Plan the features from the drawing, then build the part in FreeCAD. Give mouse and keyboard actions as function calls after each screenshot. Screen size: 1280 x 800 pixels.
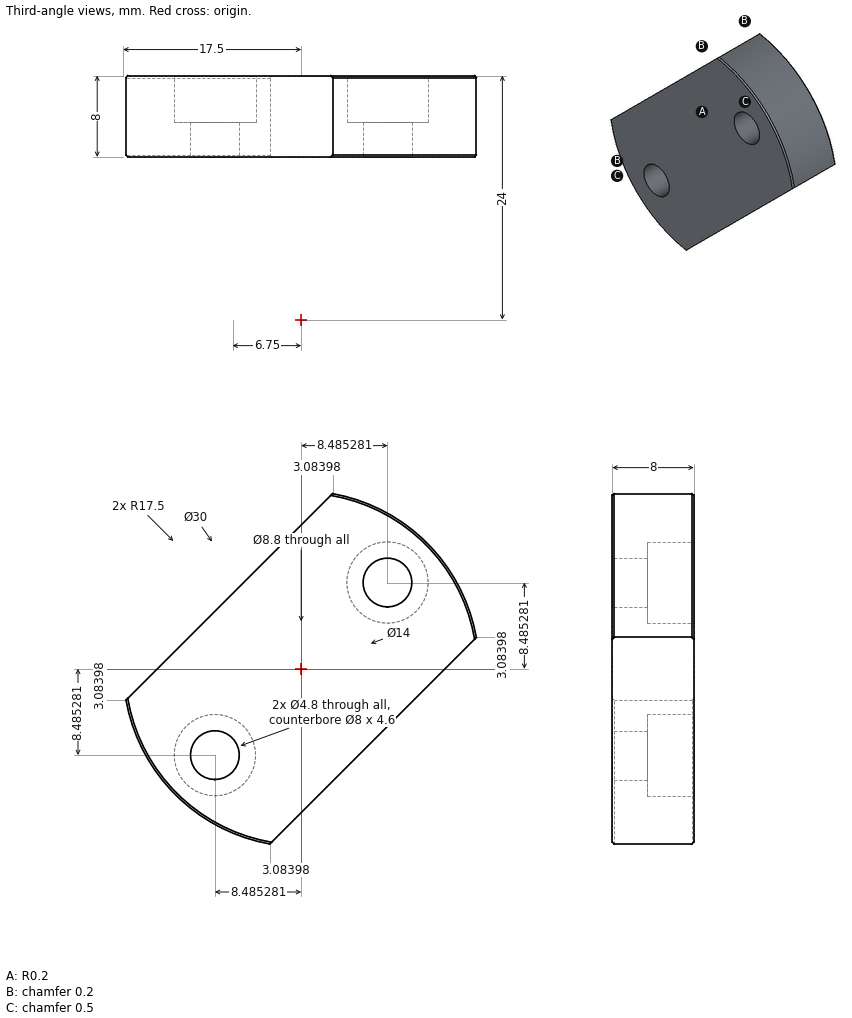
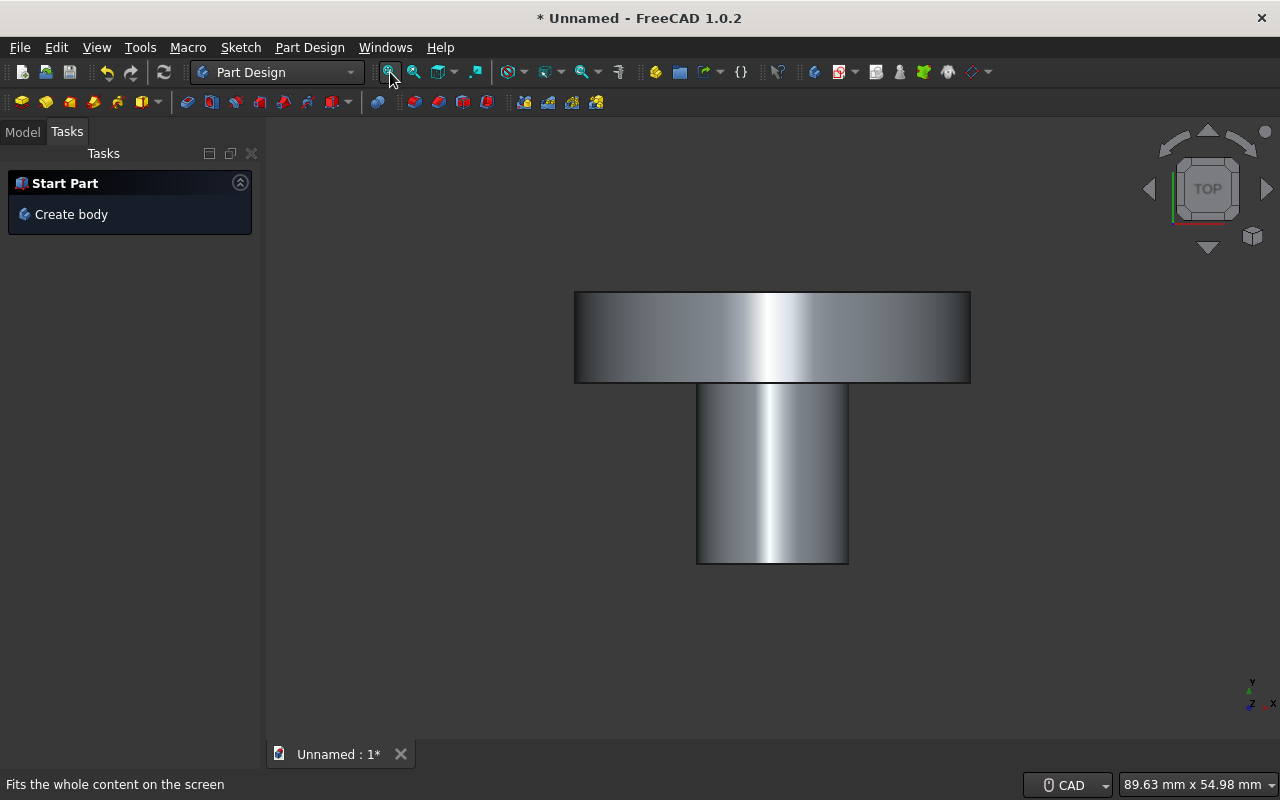
key(1)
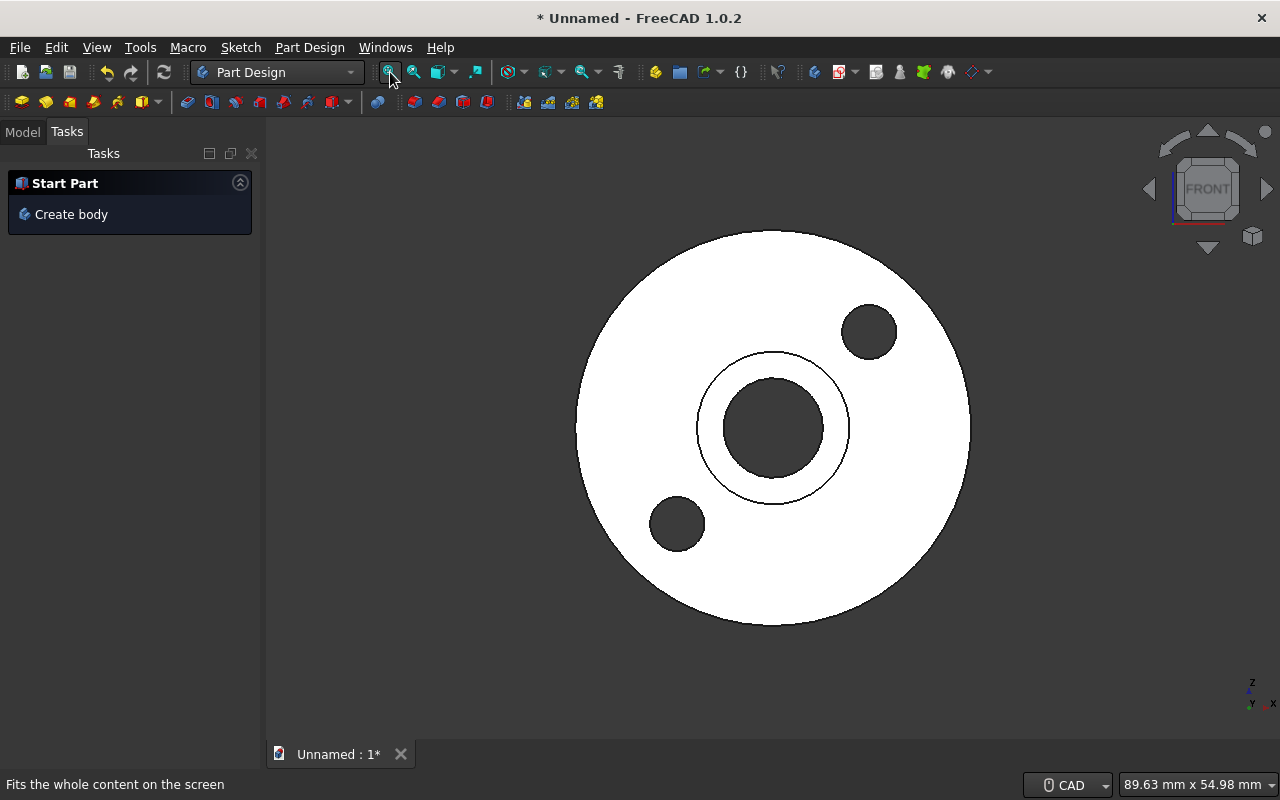
key(3)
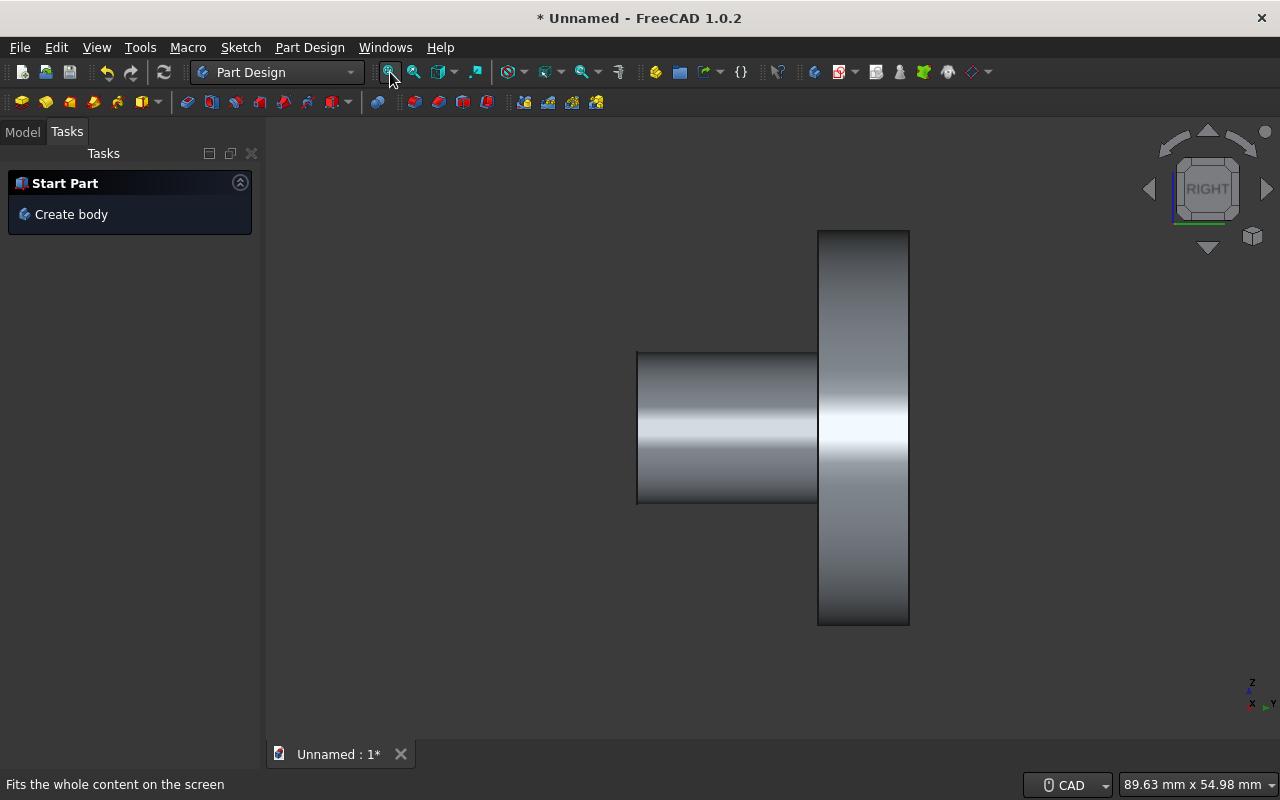
key(5)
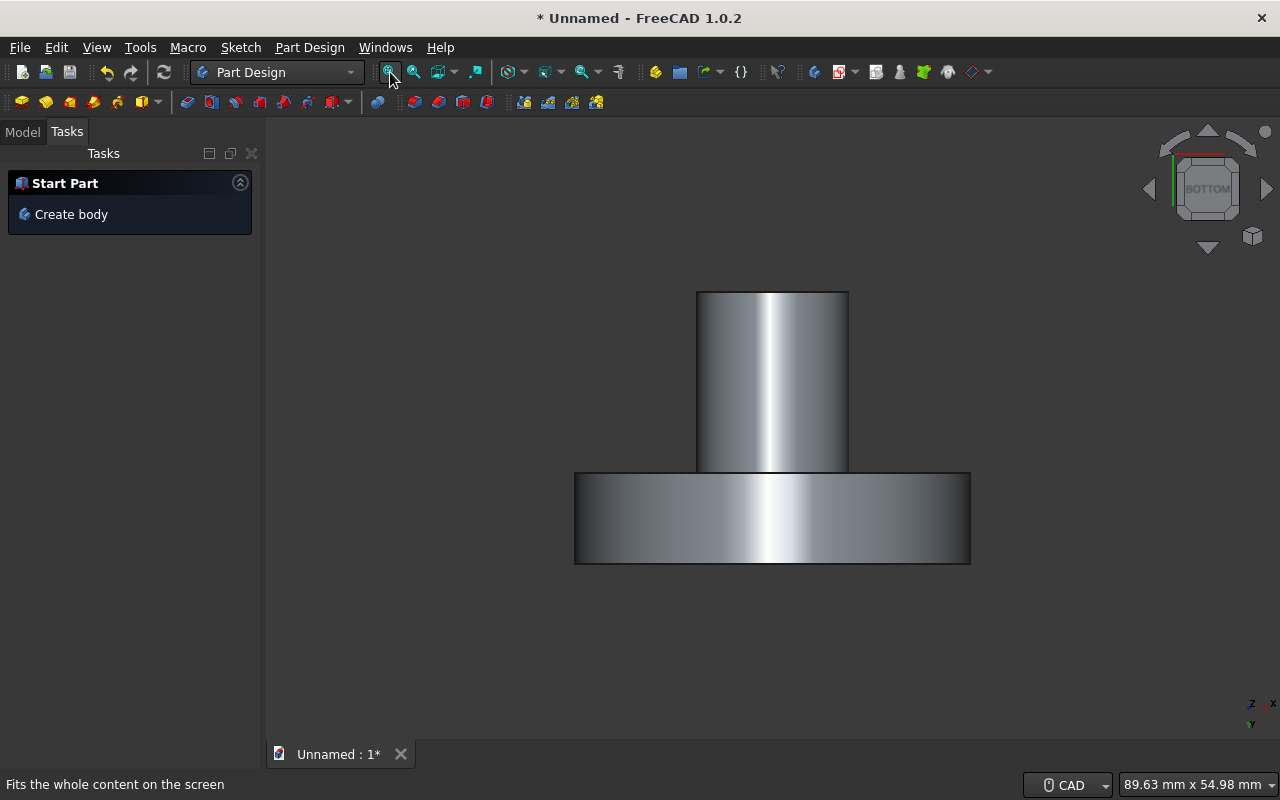
click(390, 72)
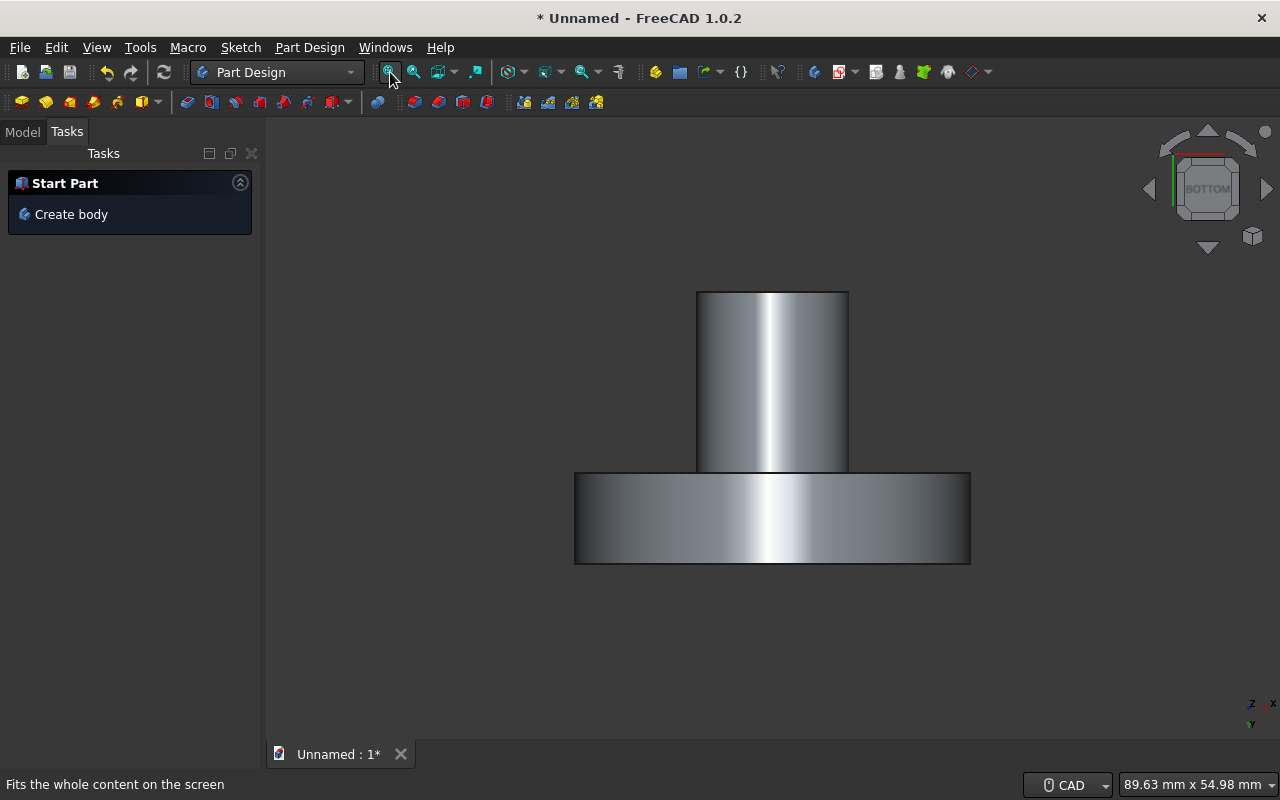
key(4)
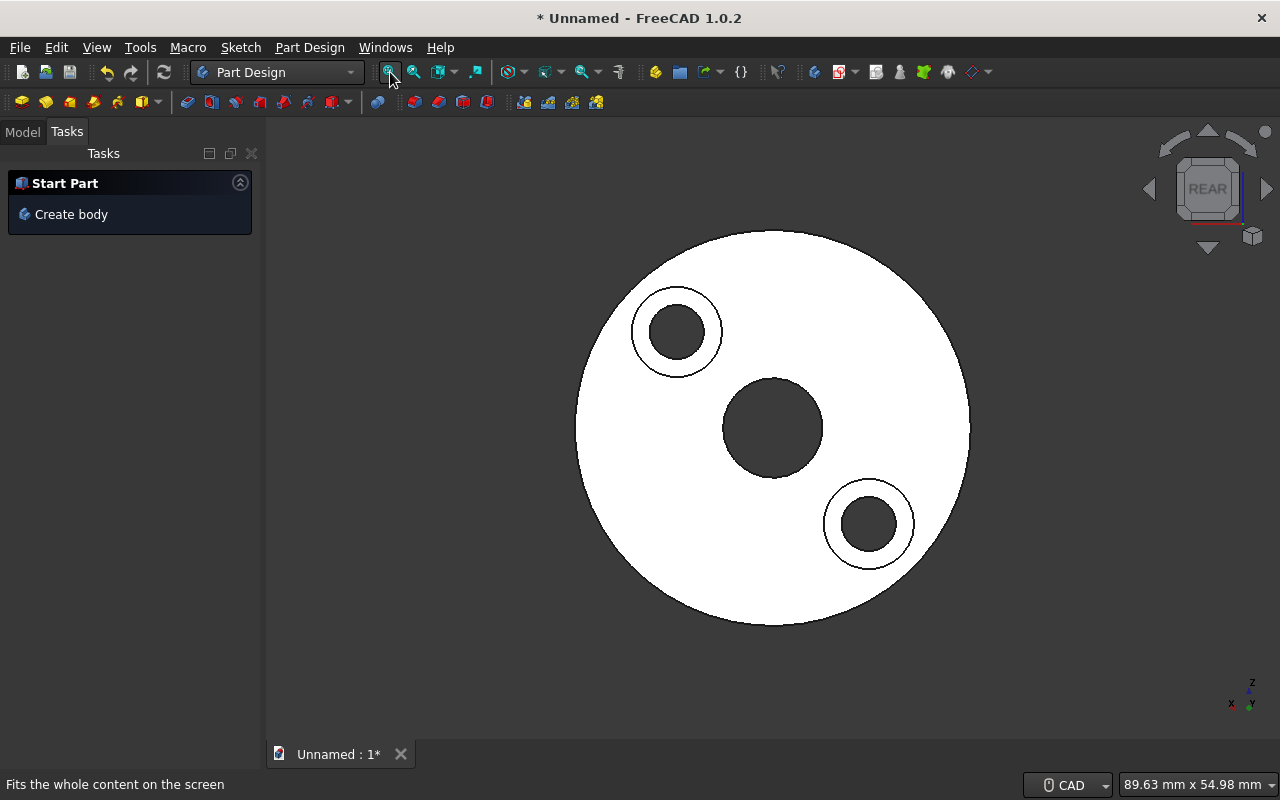
key(6)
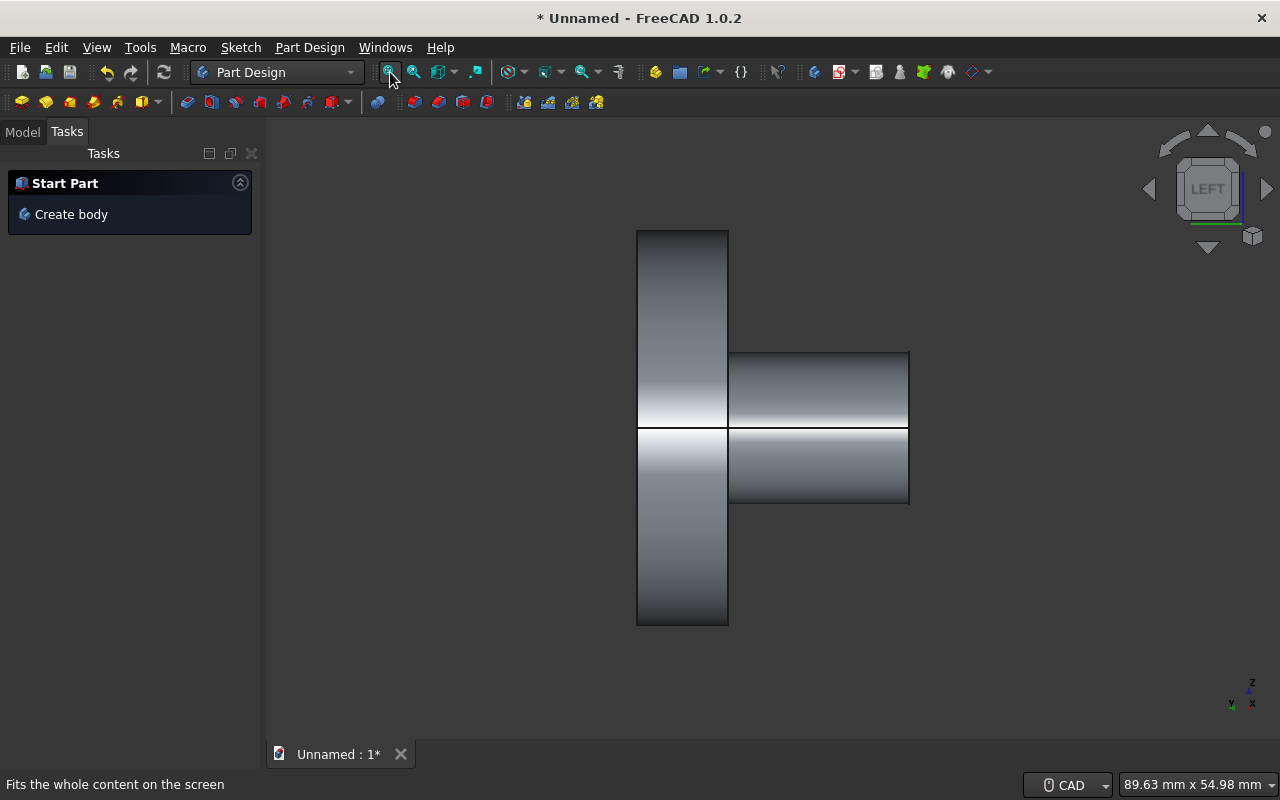
key(v)
key(3)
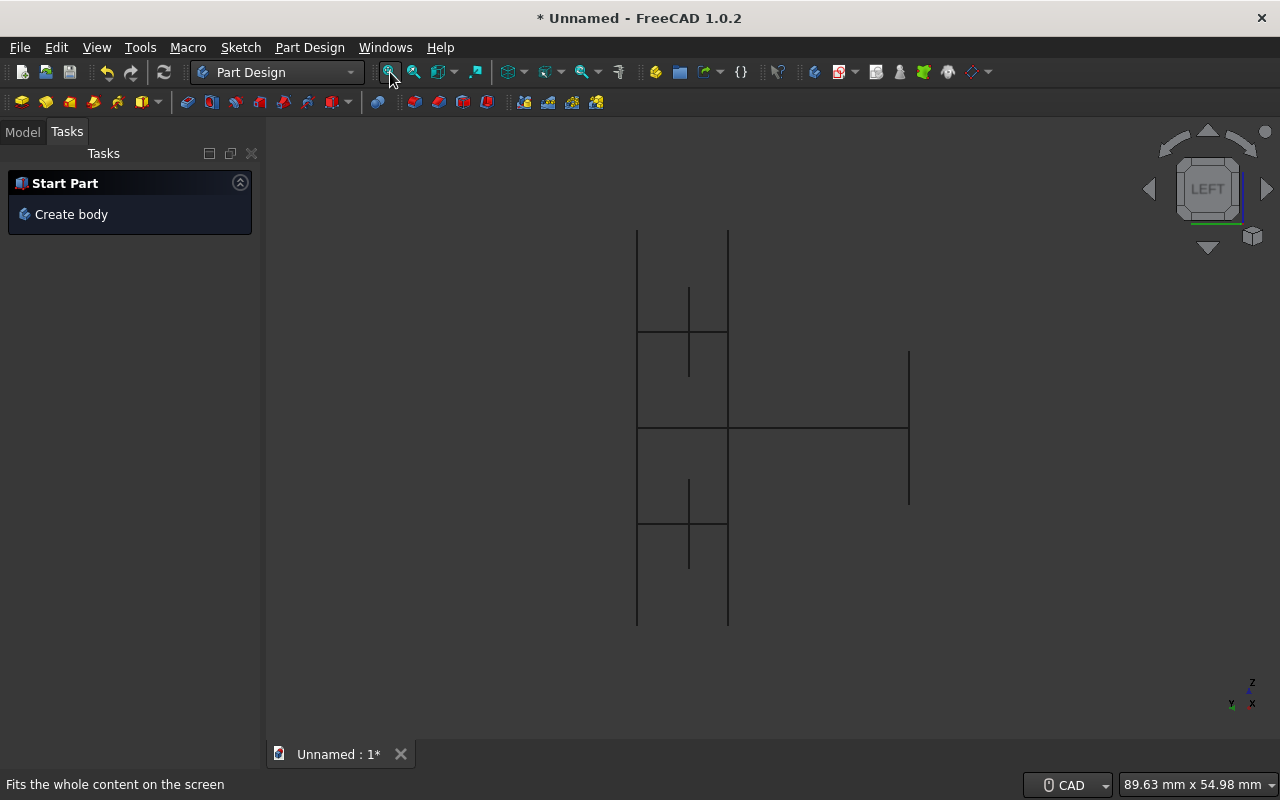
key(0)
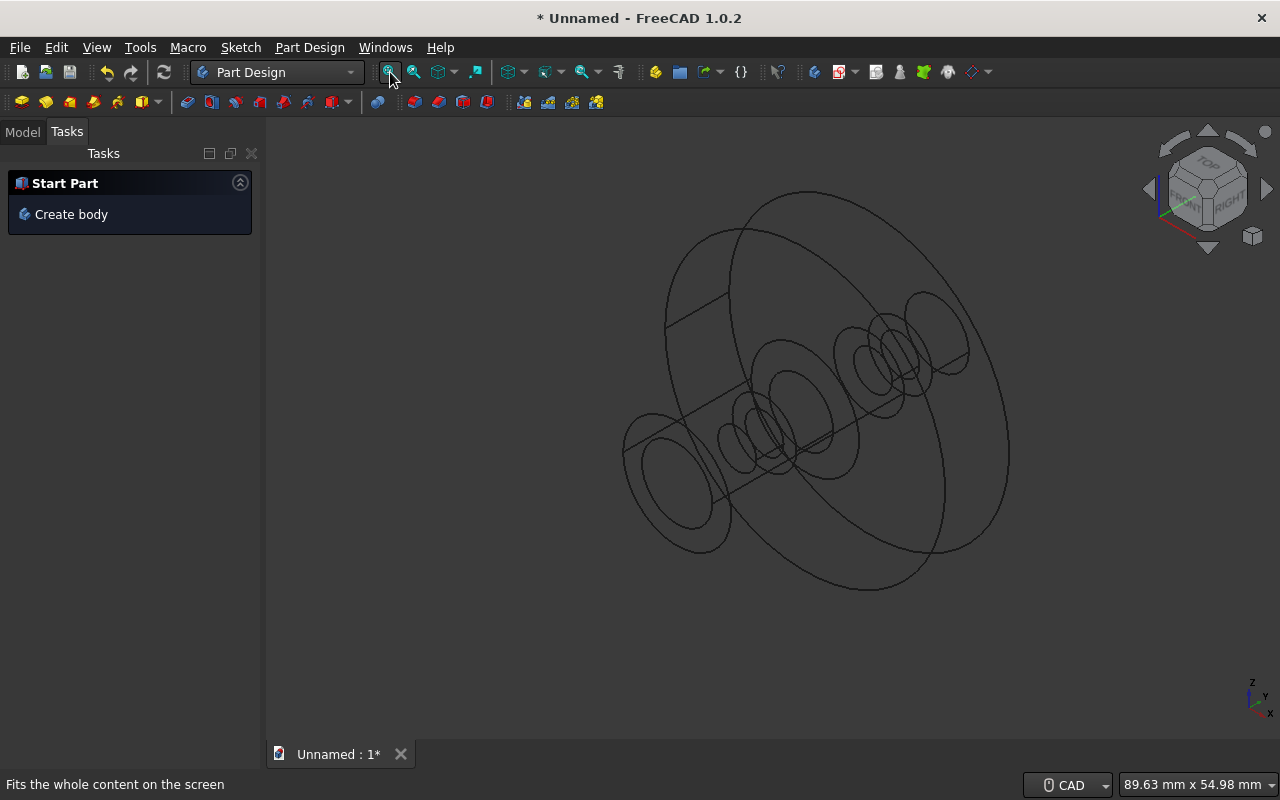
click(859, 440)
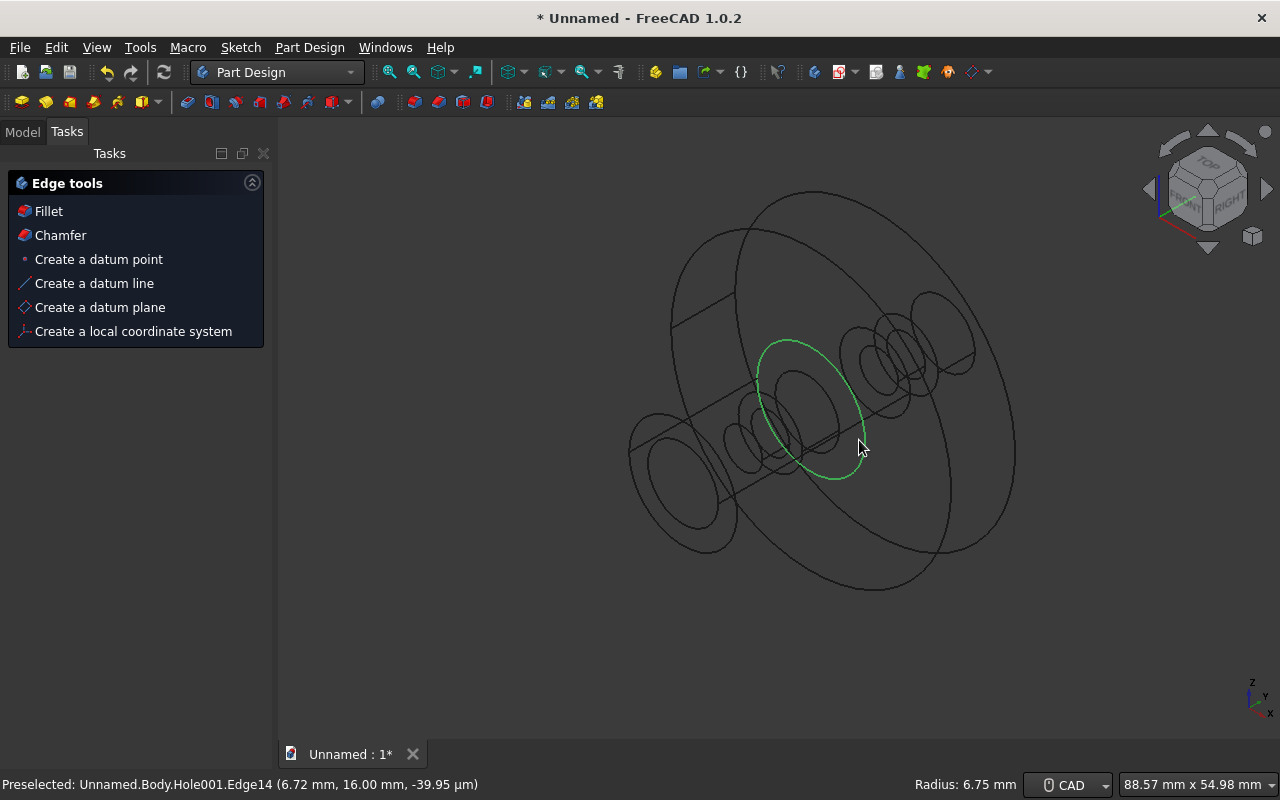
key(v)
key(1)